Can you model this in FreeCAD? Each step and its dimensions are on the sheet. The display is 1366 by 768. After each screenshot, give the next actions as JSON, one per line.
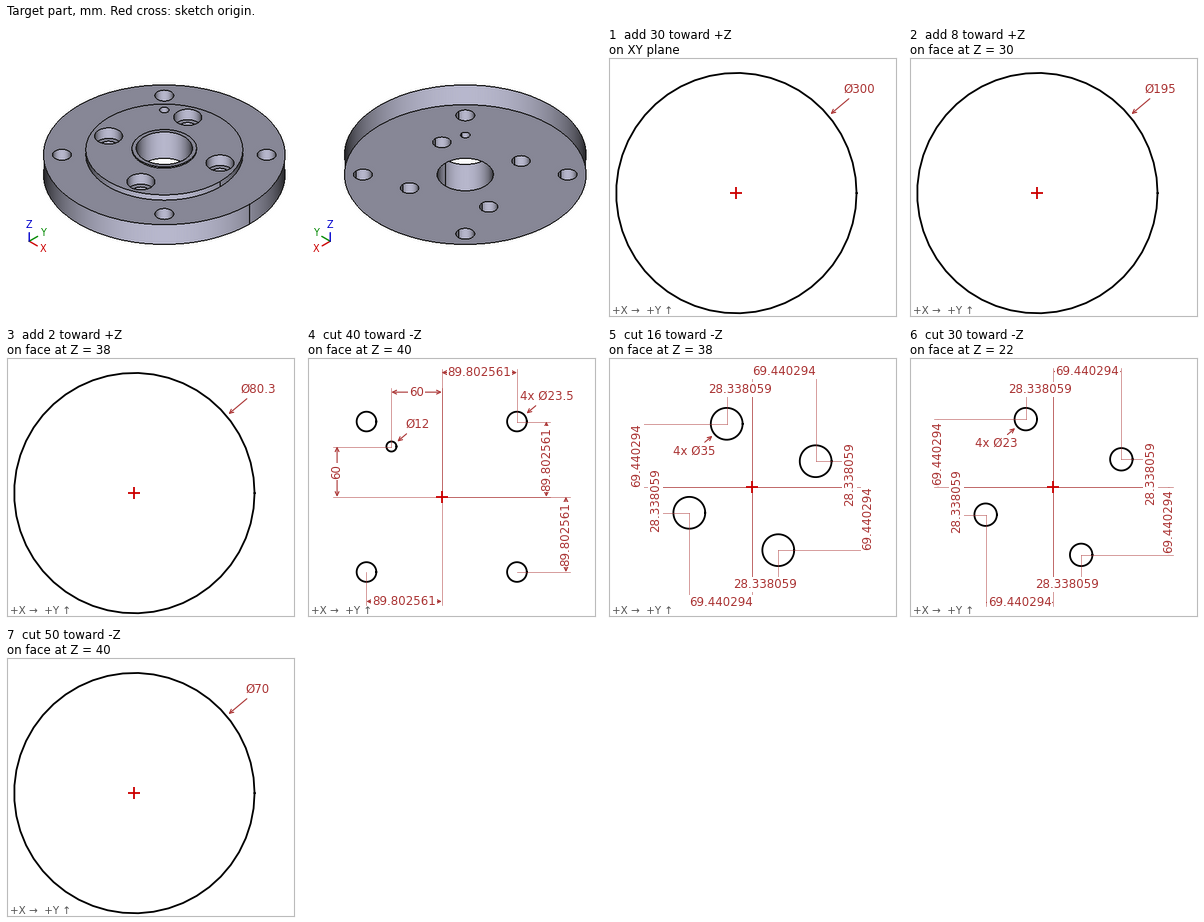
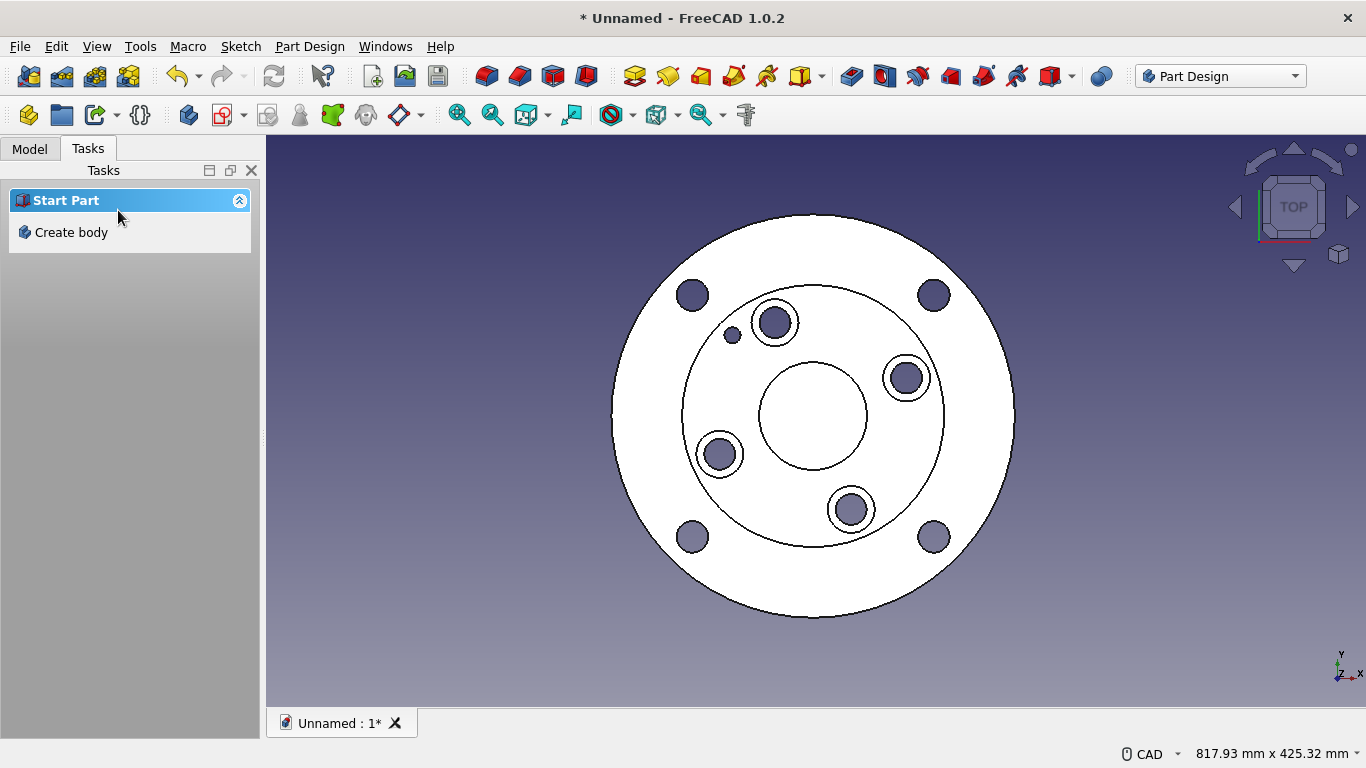
{"action": "left_click", "coordinate": [813, 415]}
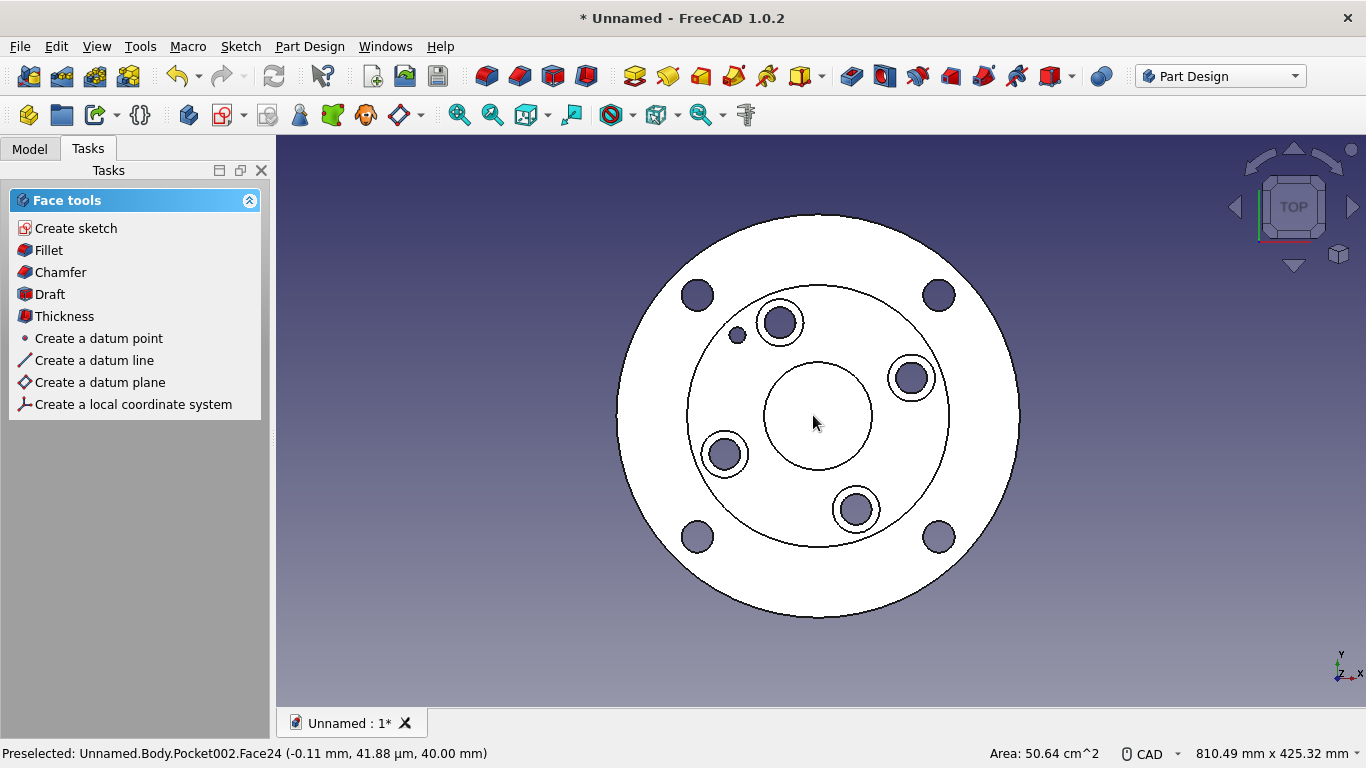
{"action": "left_click", "coordinate": [222, 116]}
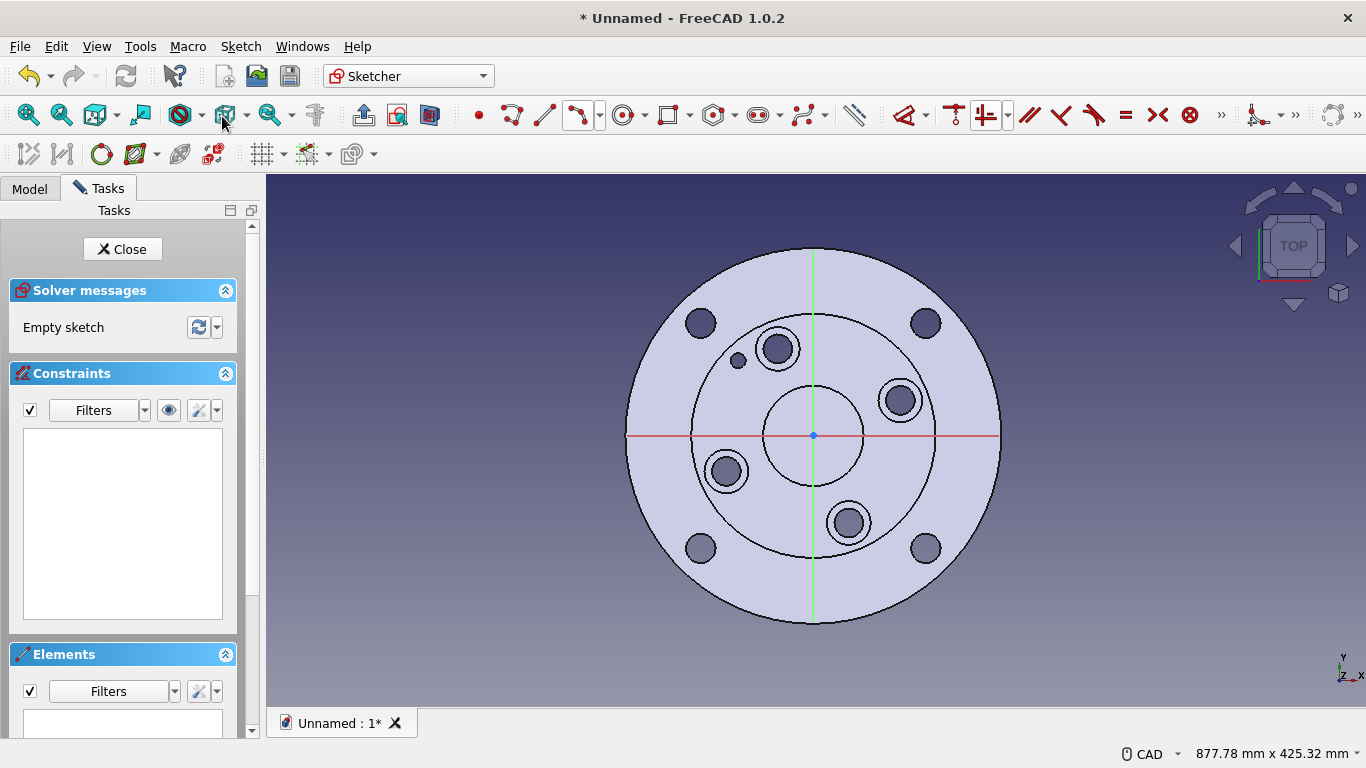
{"action": "scroll", "coordinate": [835, 434], "scroll_direction": "up", "scroll_amount": 7}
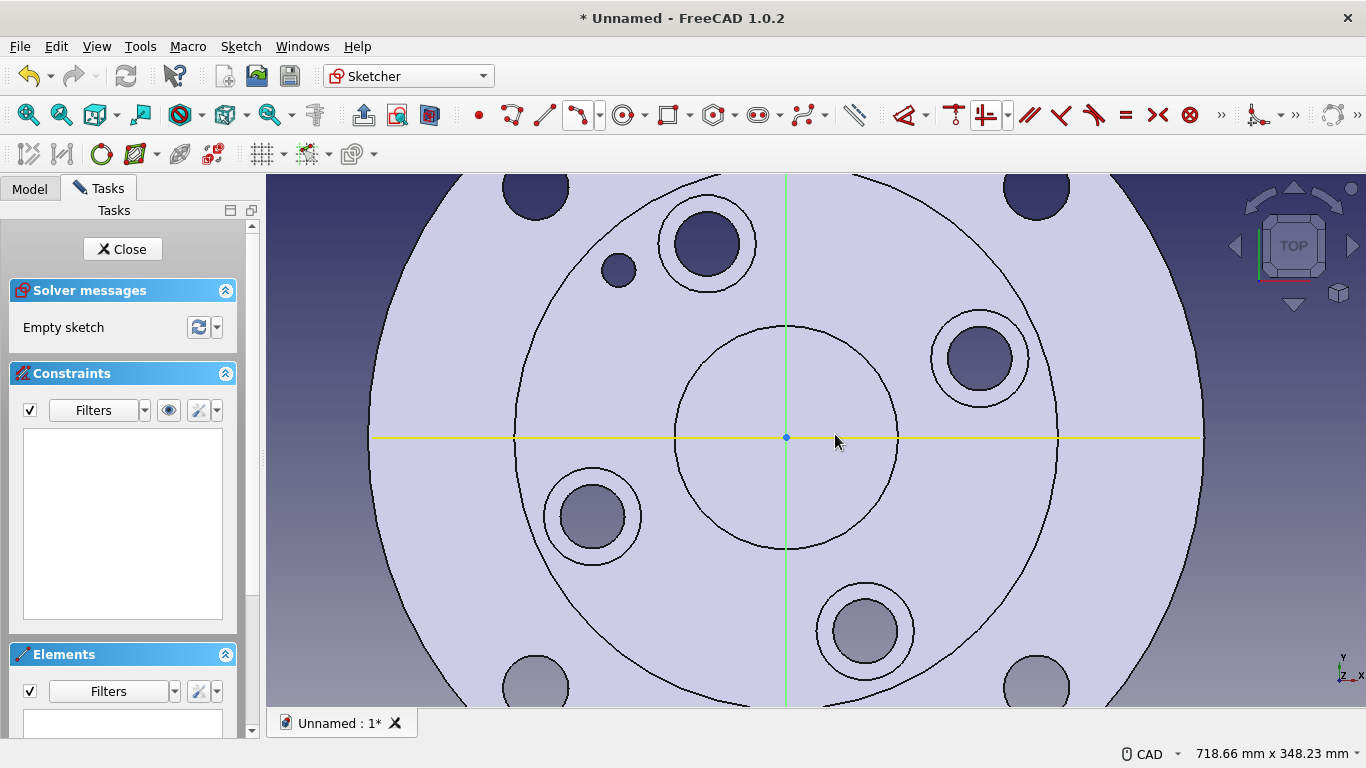
{"action": "left_click", "coordinate": [622, 116]}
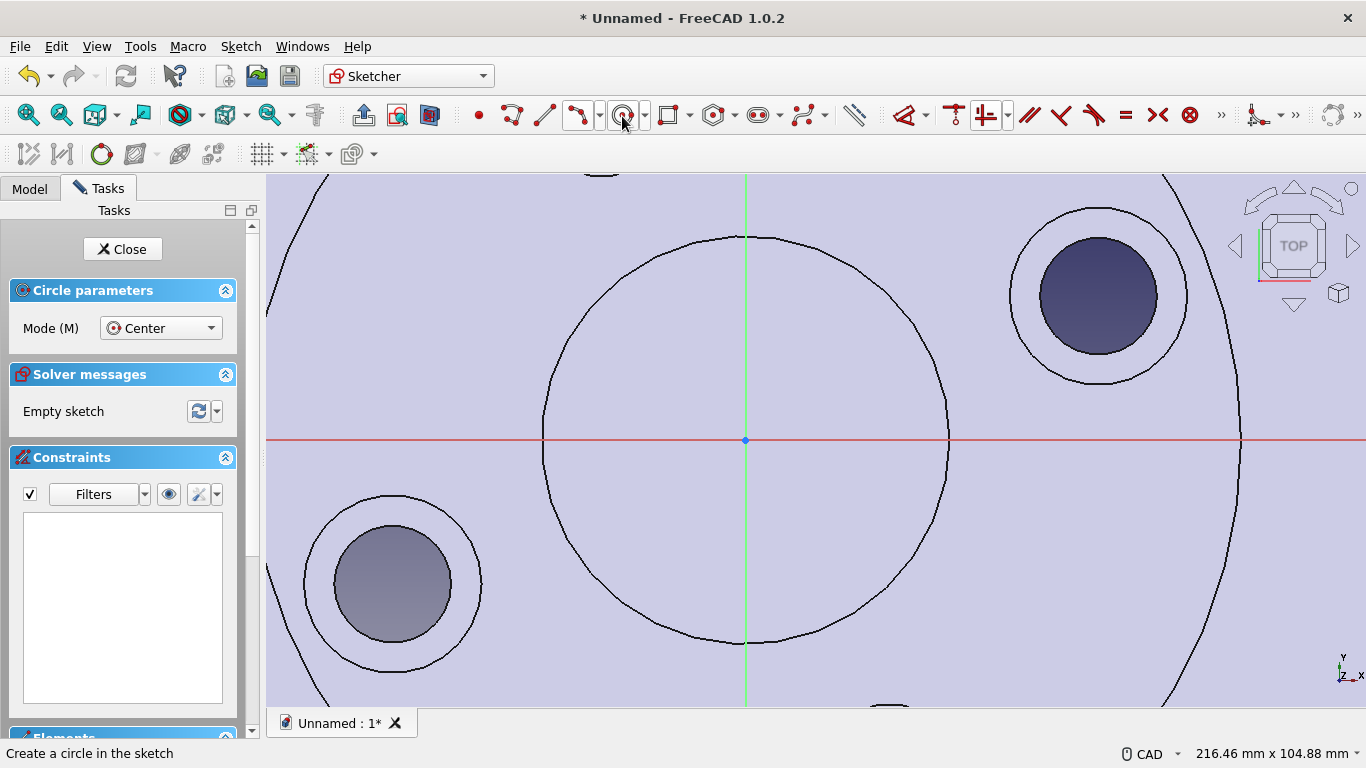
{"action": "left_click", "coordinate": [746, 440]}
{"action": "left_click", "coordinate": [871, 314]}
{"action": "key", "text": "Escape"}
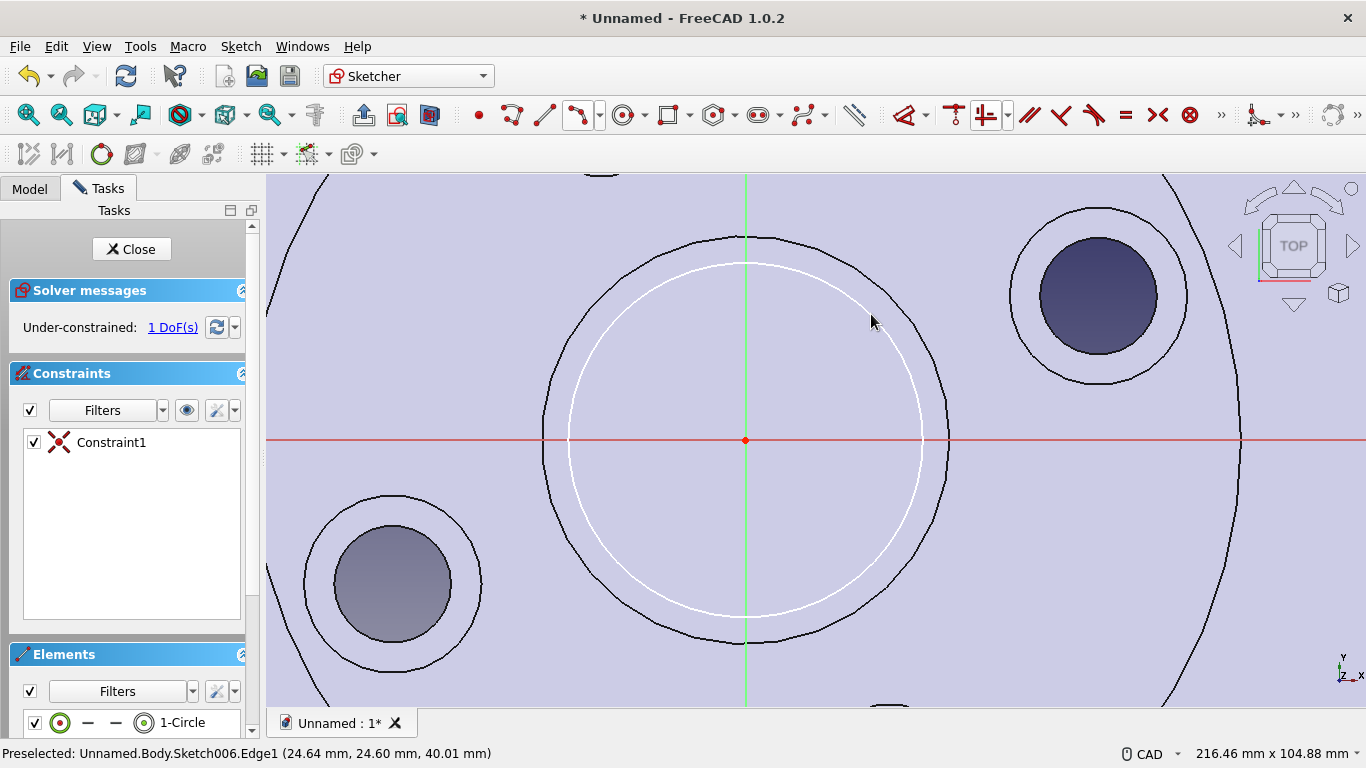
{"action": "left_click", "coordinate": [904, 116]}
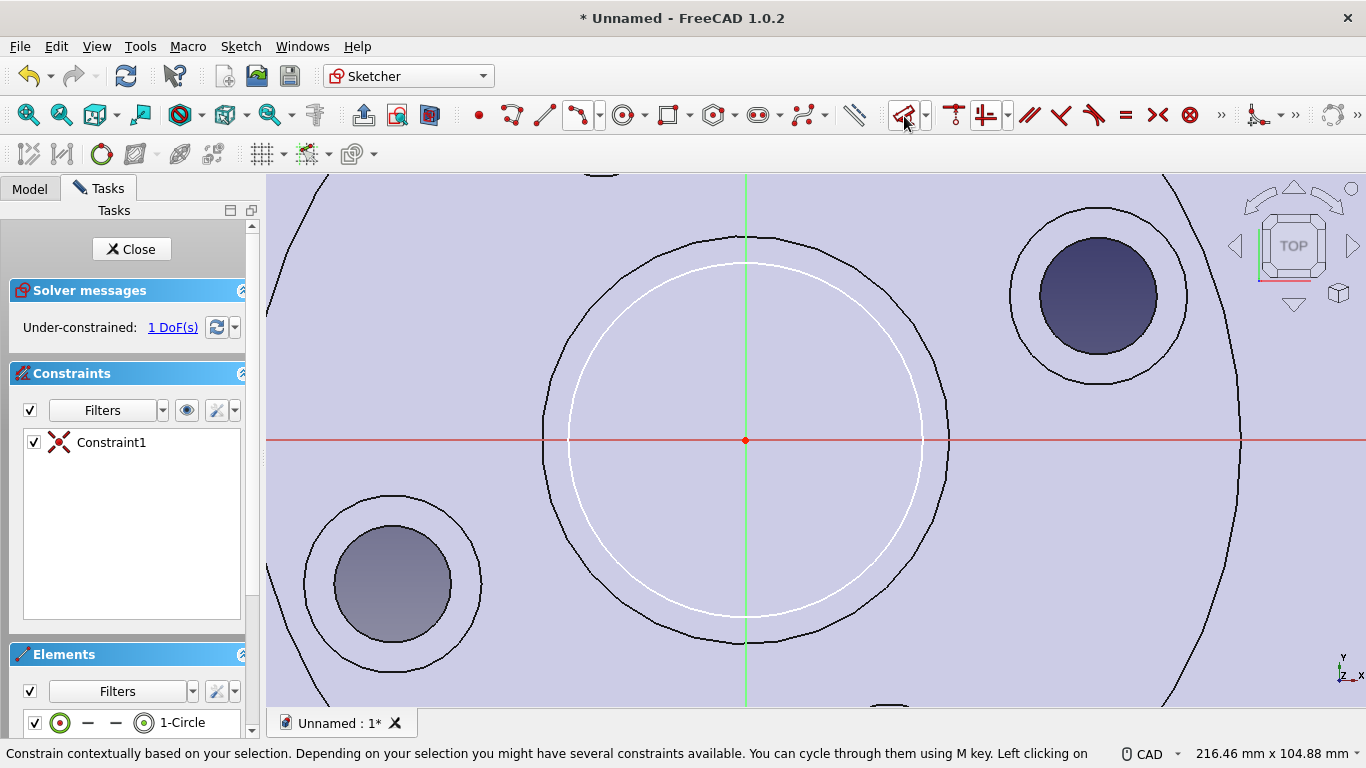
{"action": "left_click", "coordinate": [870, 314]}
{"action": "left_click", "coordinate": [892, 291]}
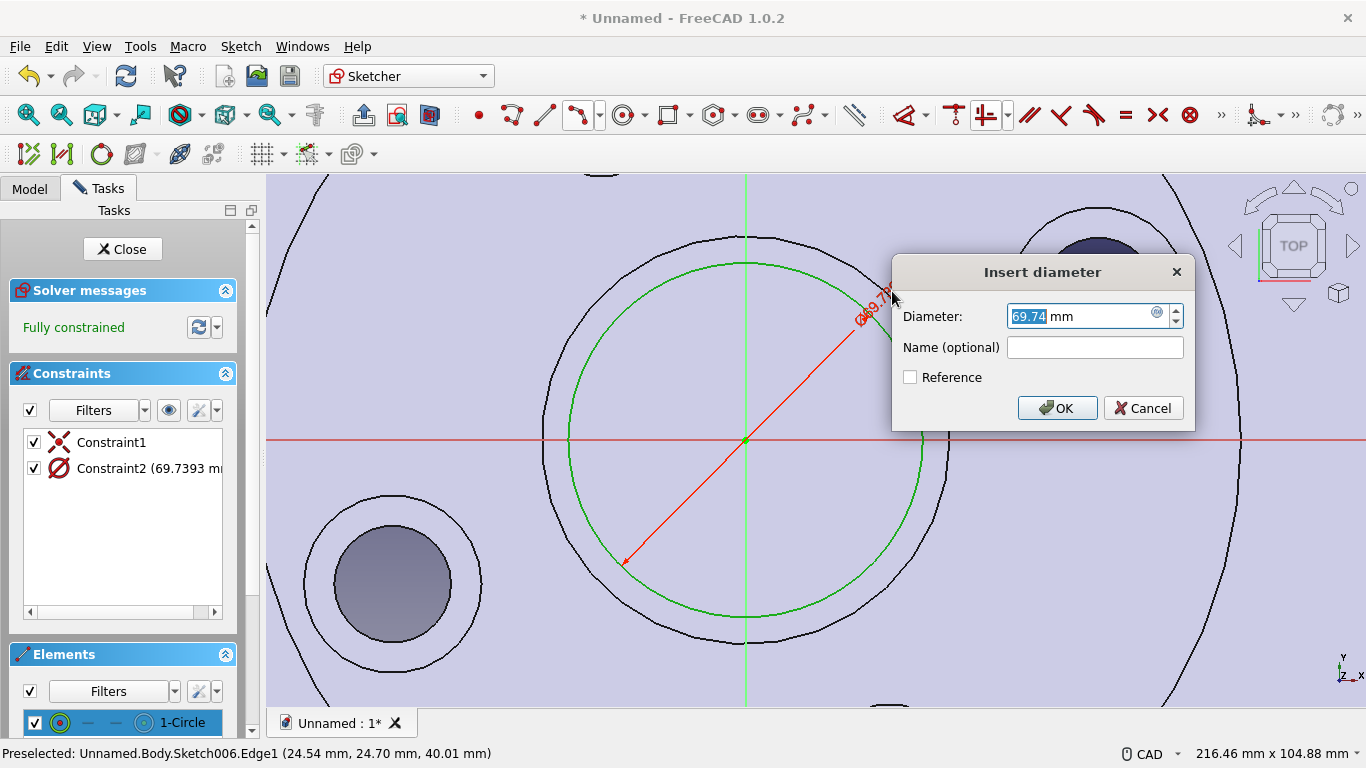
{"action": "type", "text": "70"}
{"action": "key", "text": "Return"}
{"action": "key", "text": "Escape"}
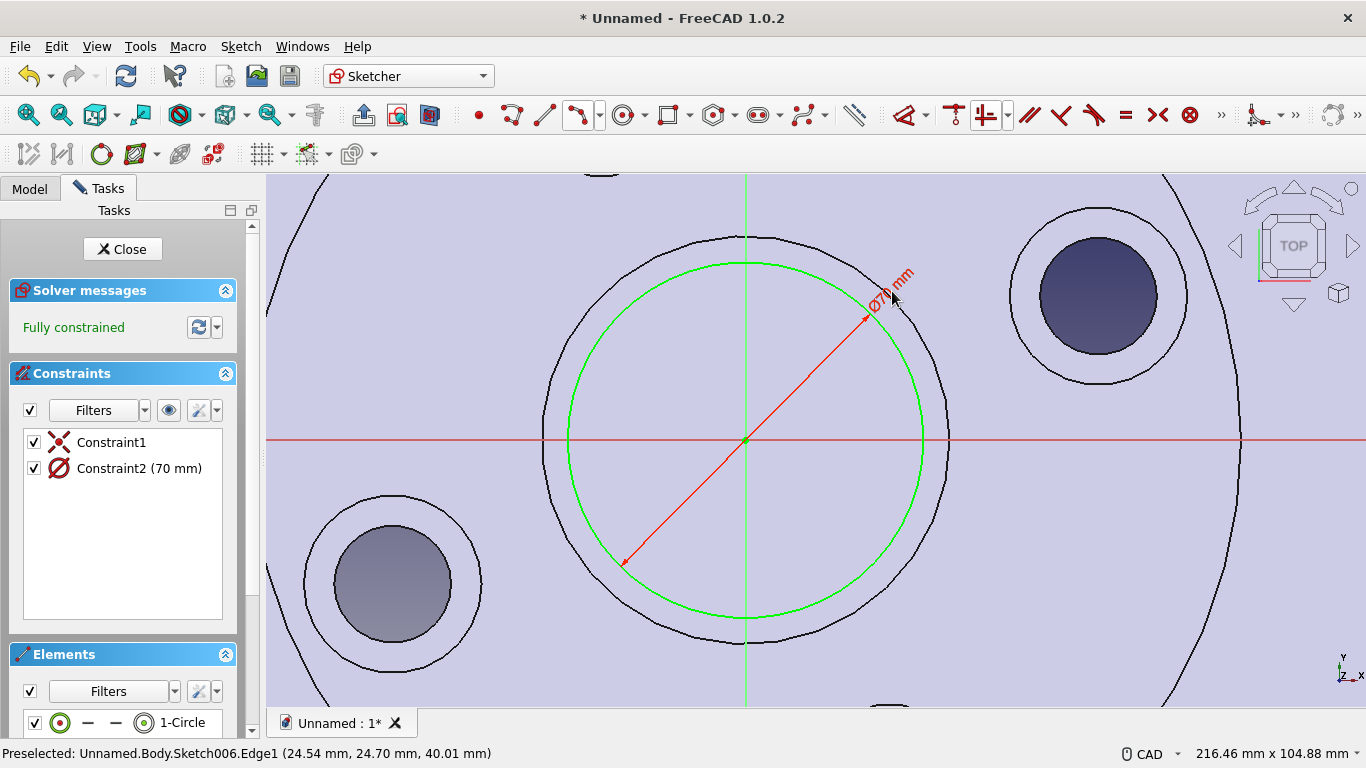
{"action": "left_click", "coordinate": [123, 249]}